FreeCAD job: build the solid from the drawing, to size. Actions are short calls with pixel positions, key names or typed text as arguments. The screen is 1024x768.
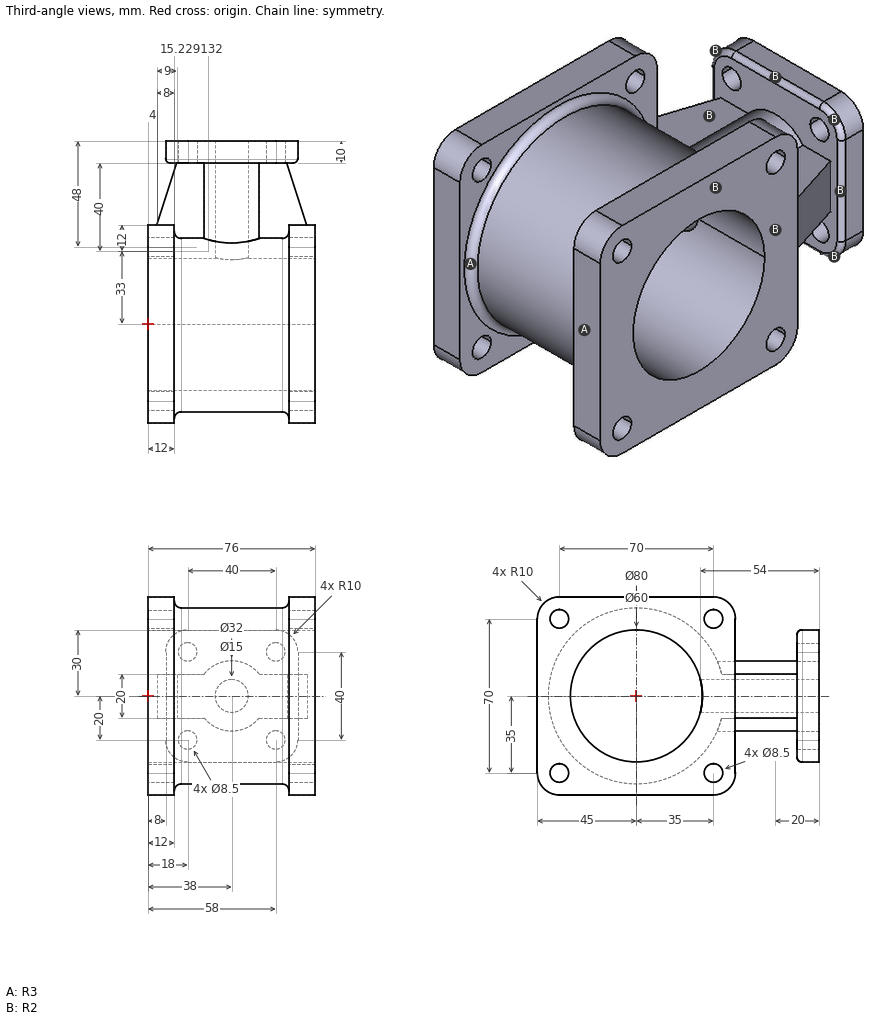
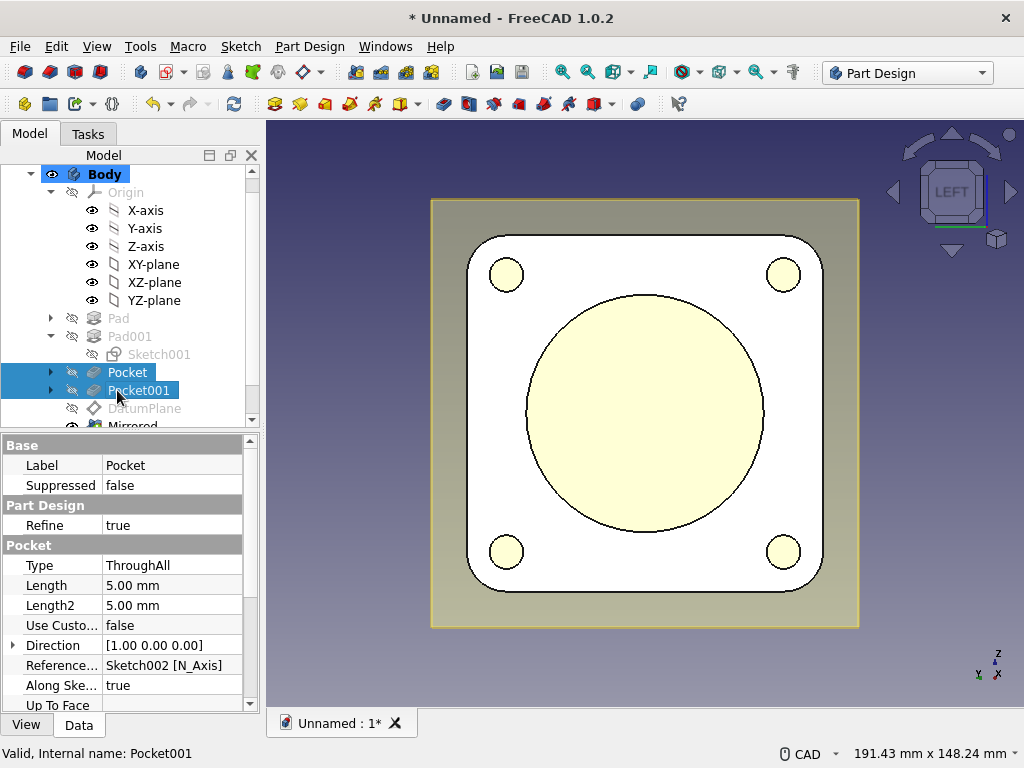
click(356, 72)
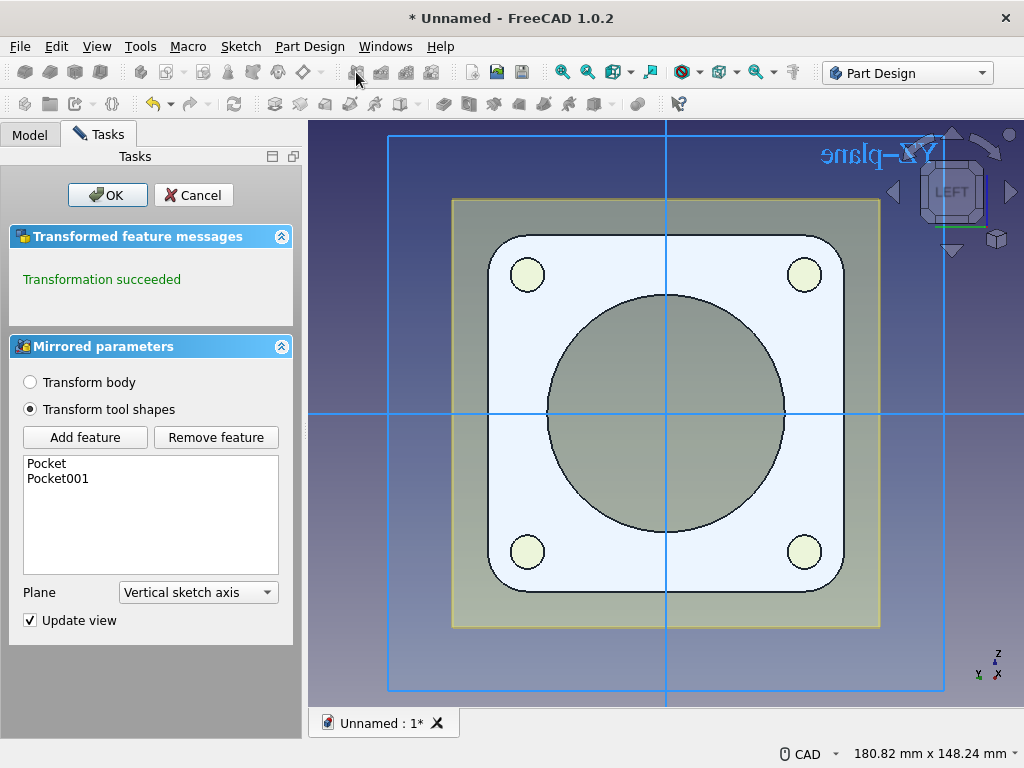
click(199, 592)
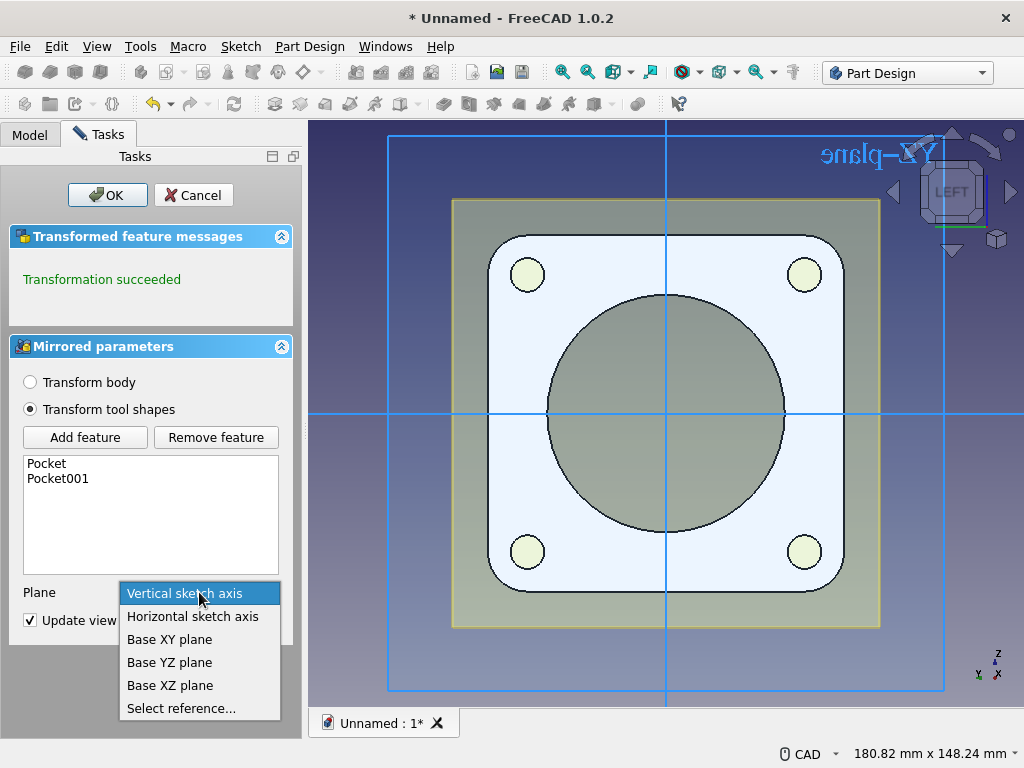
click(198, 708)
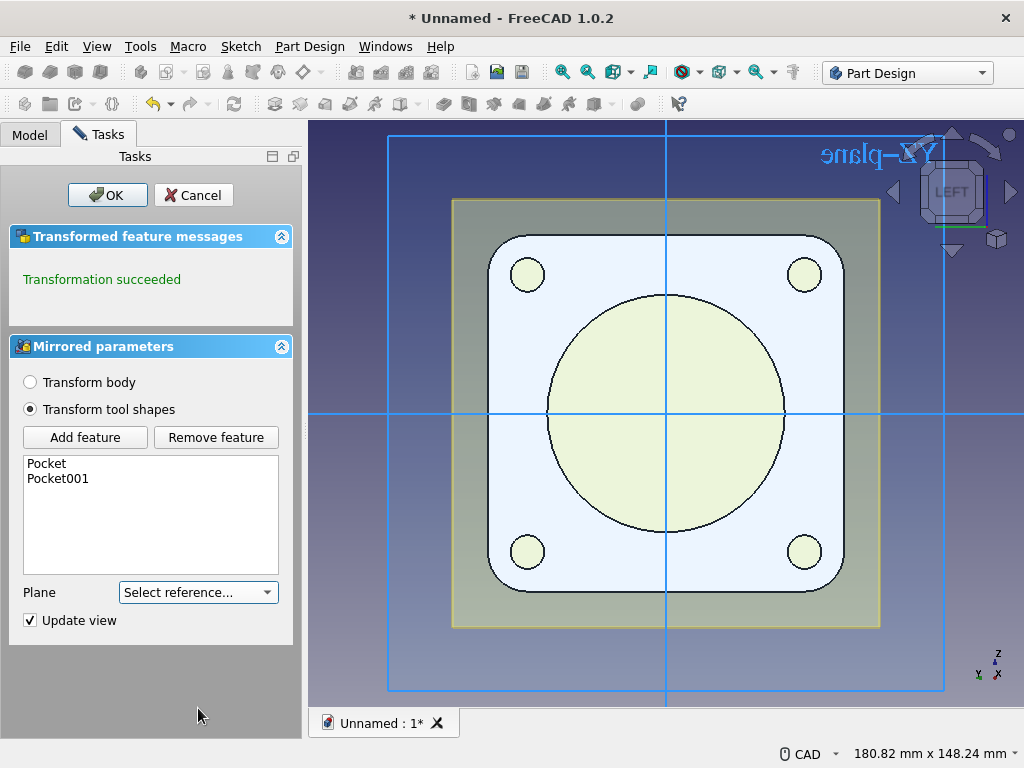
click(30, 134)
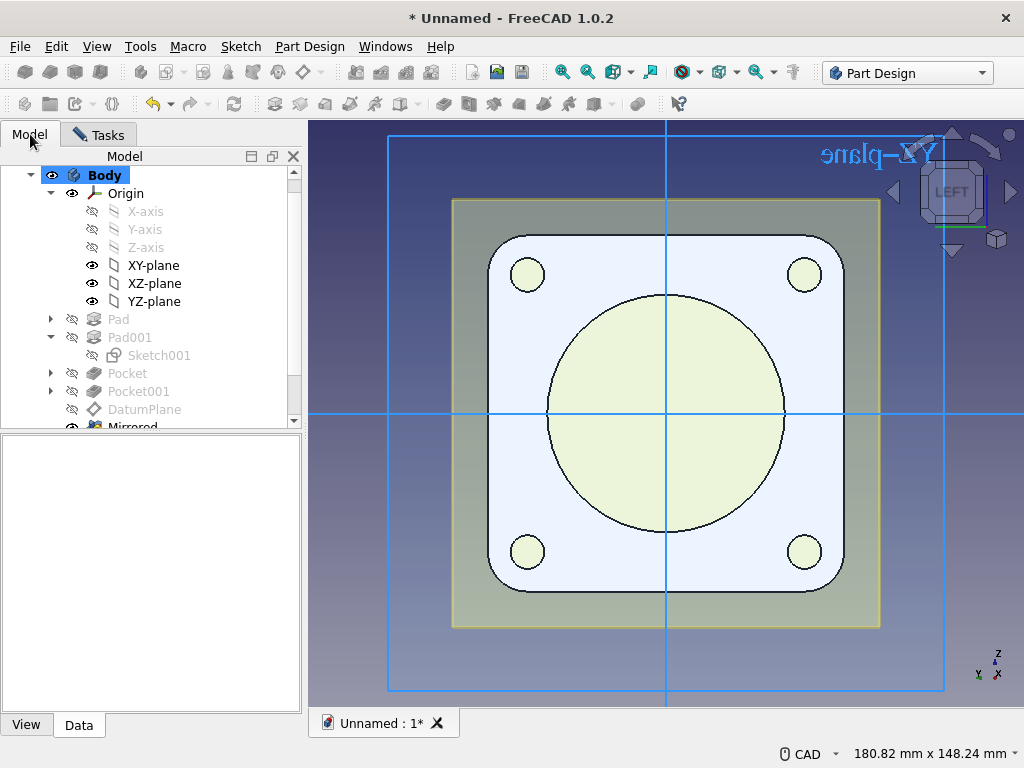
scroll(121, 297, down, 3)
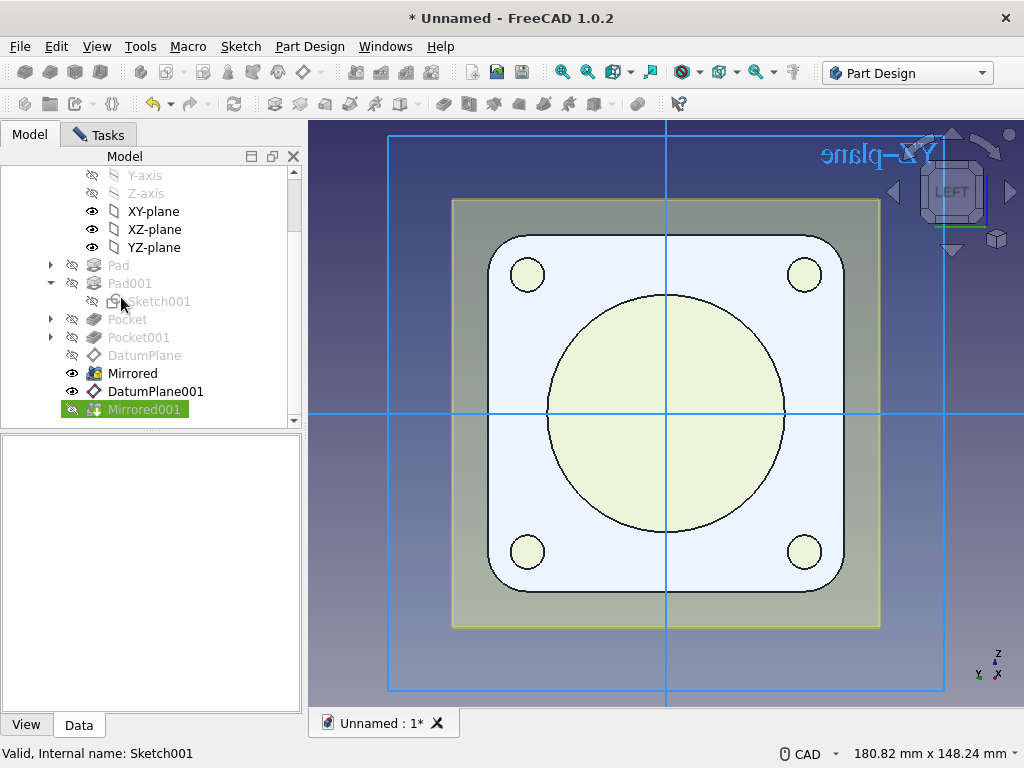
click(117, 391)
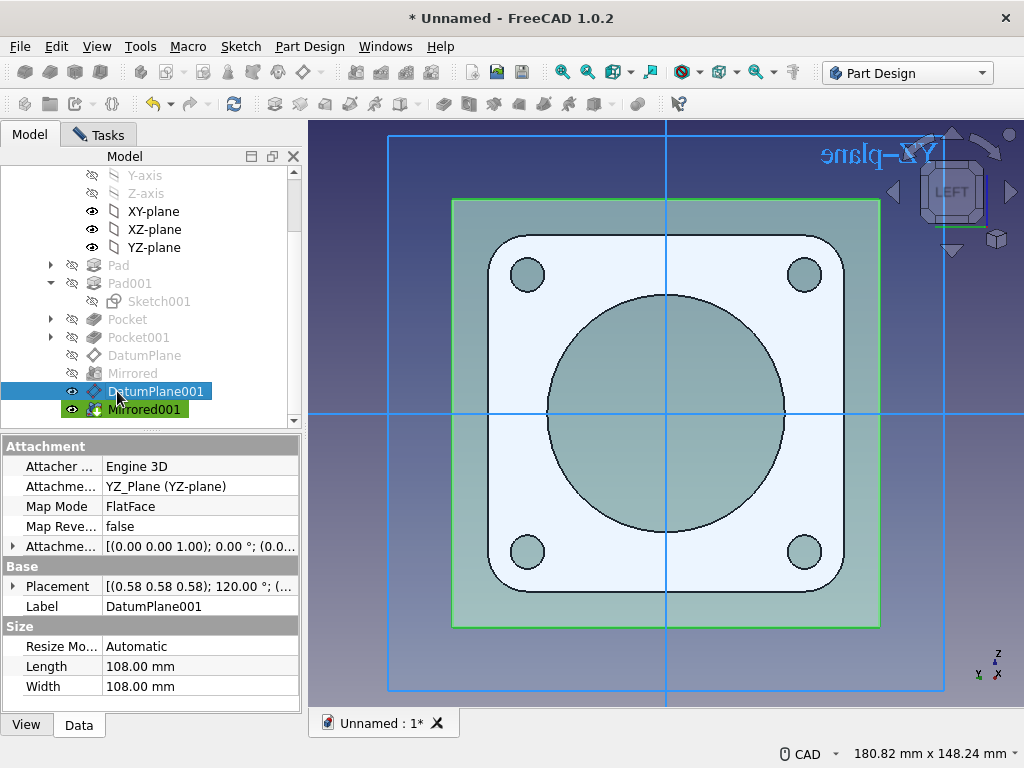
click(98, 134)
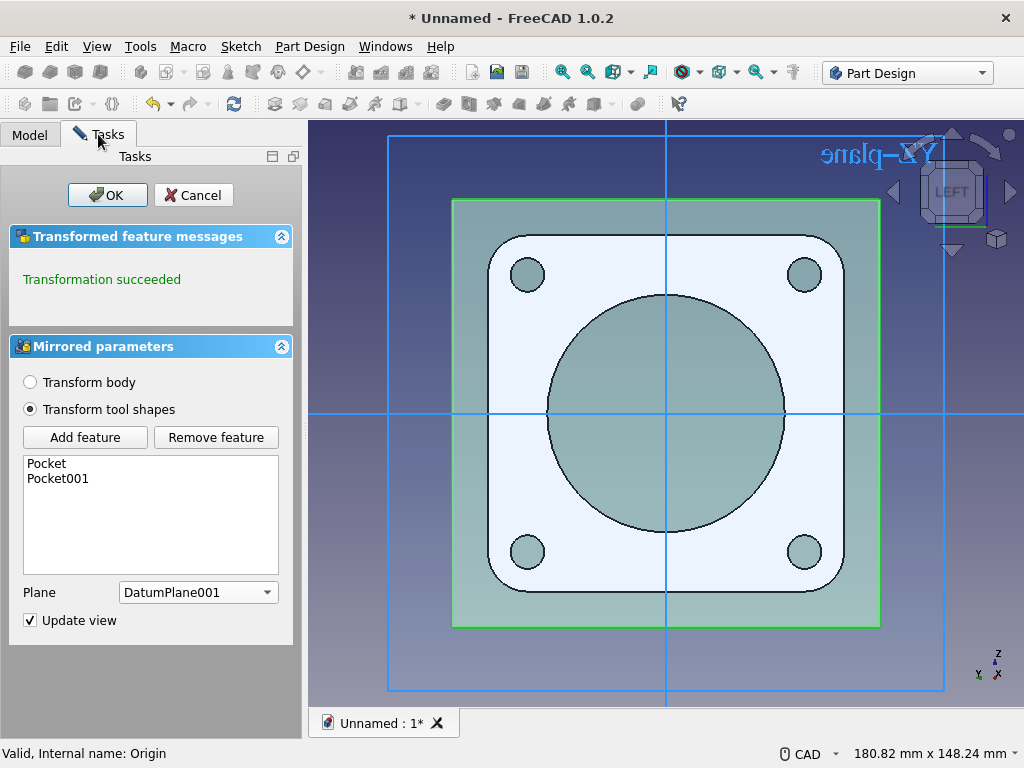
click(108, 195)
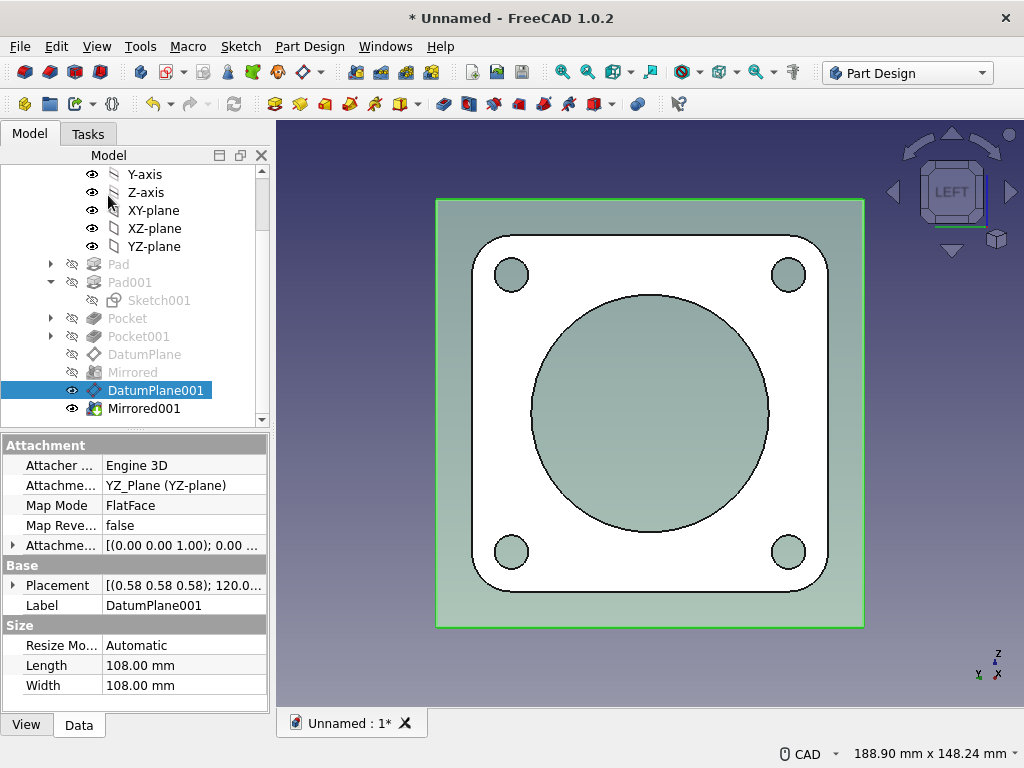
click(117, 390)
key(space)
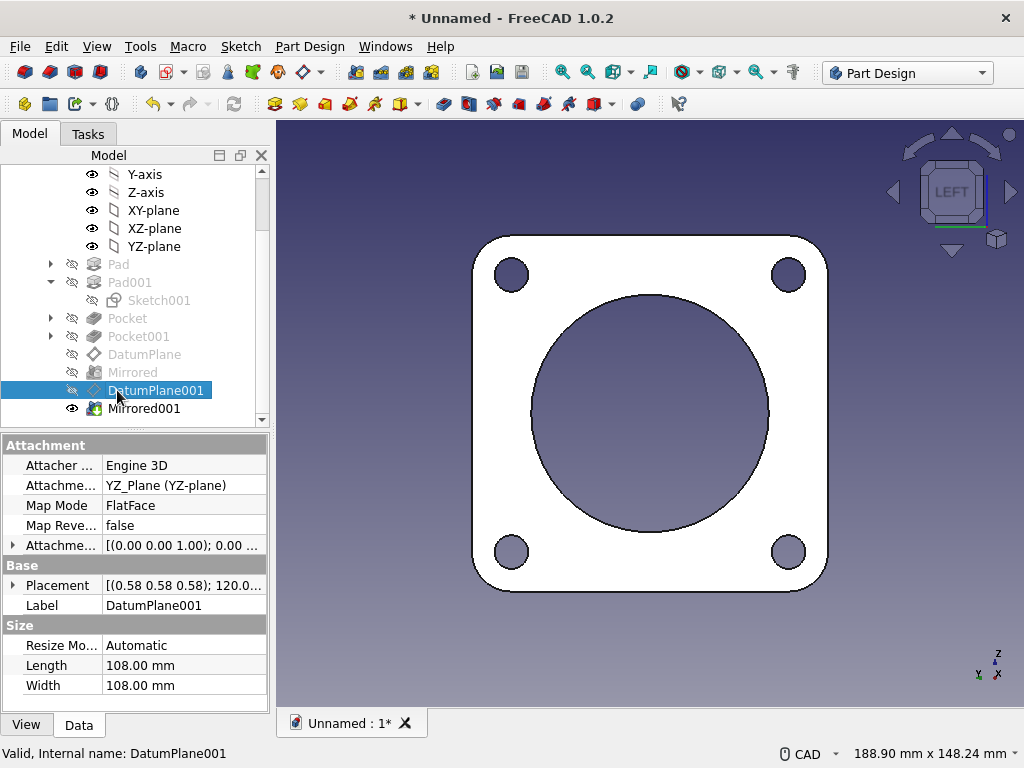
click(316, 667)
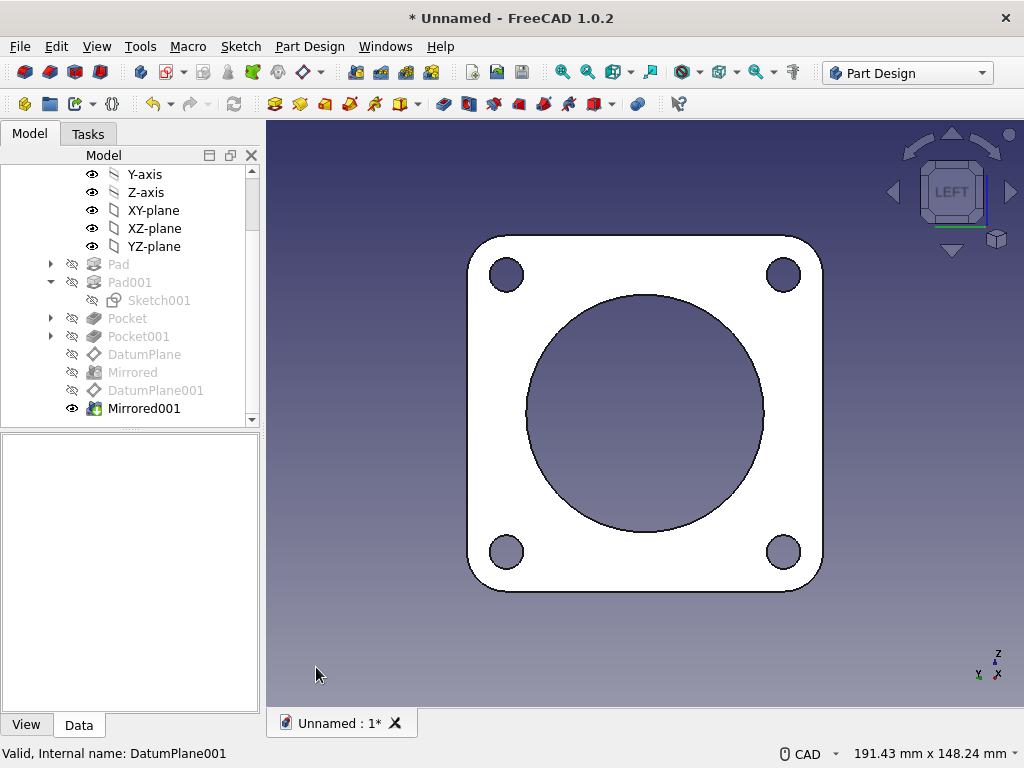
click(141, 72)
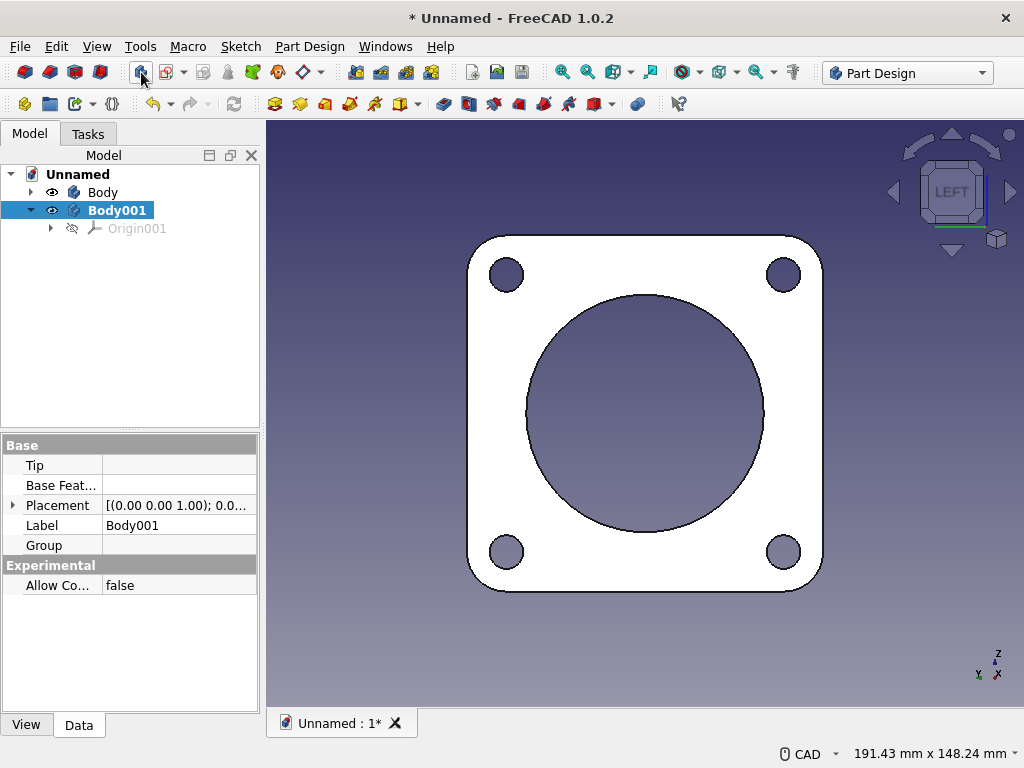
click(51, 228)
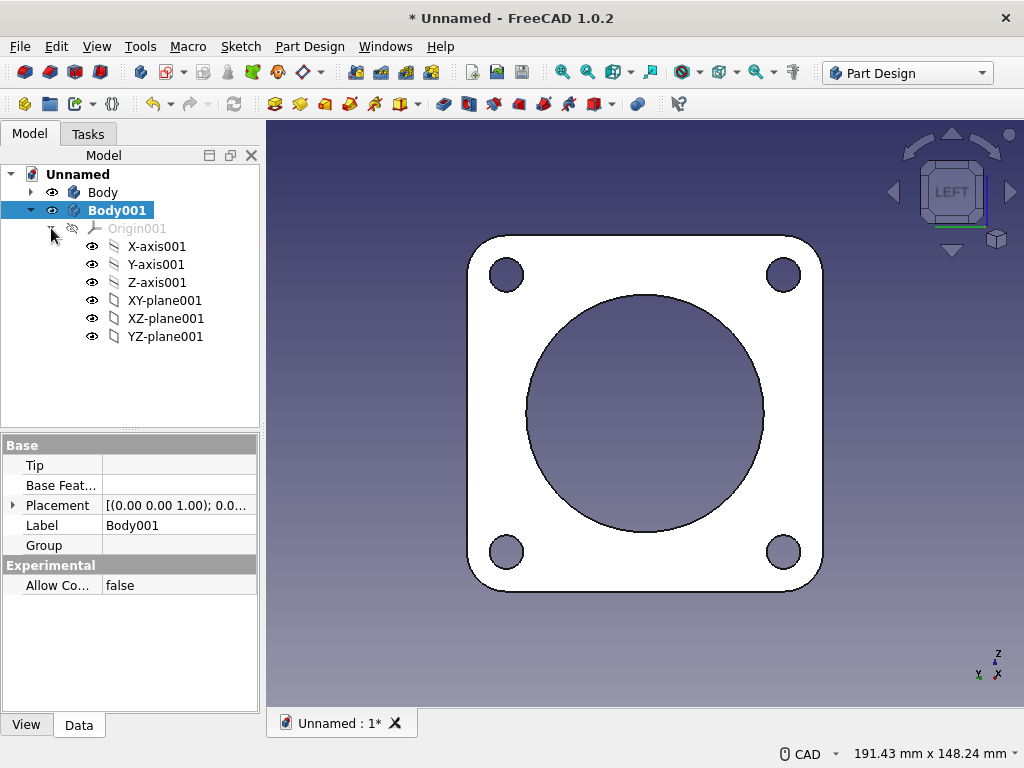
click(137, 318)